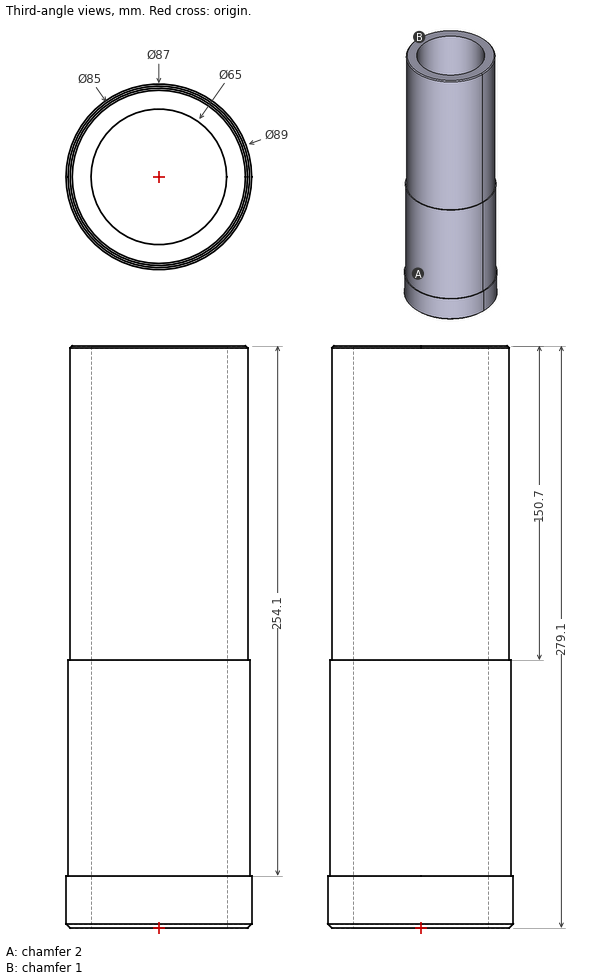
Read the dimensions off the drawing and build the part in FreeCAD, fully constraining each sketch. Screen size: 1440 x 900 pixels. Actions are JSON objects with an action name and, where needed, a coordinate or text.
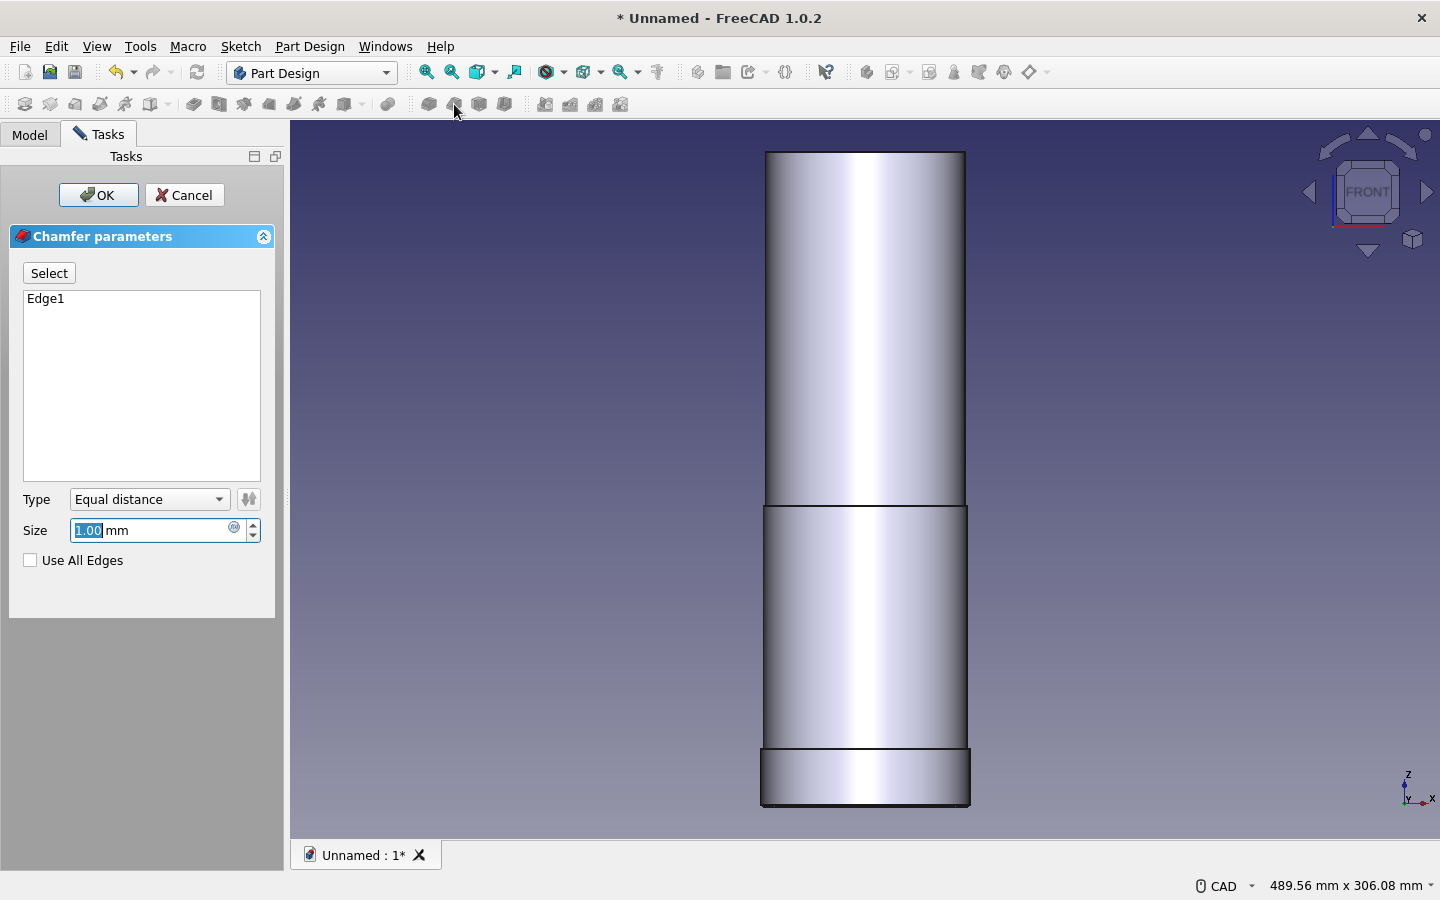
{"action": "type", "text": "2"}
{"action": "key", "text": "Tab"}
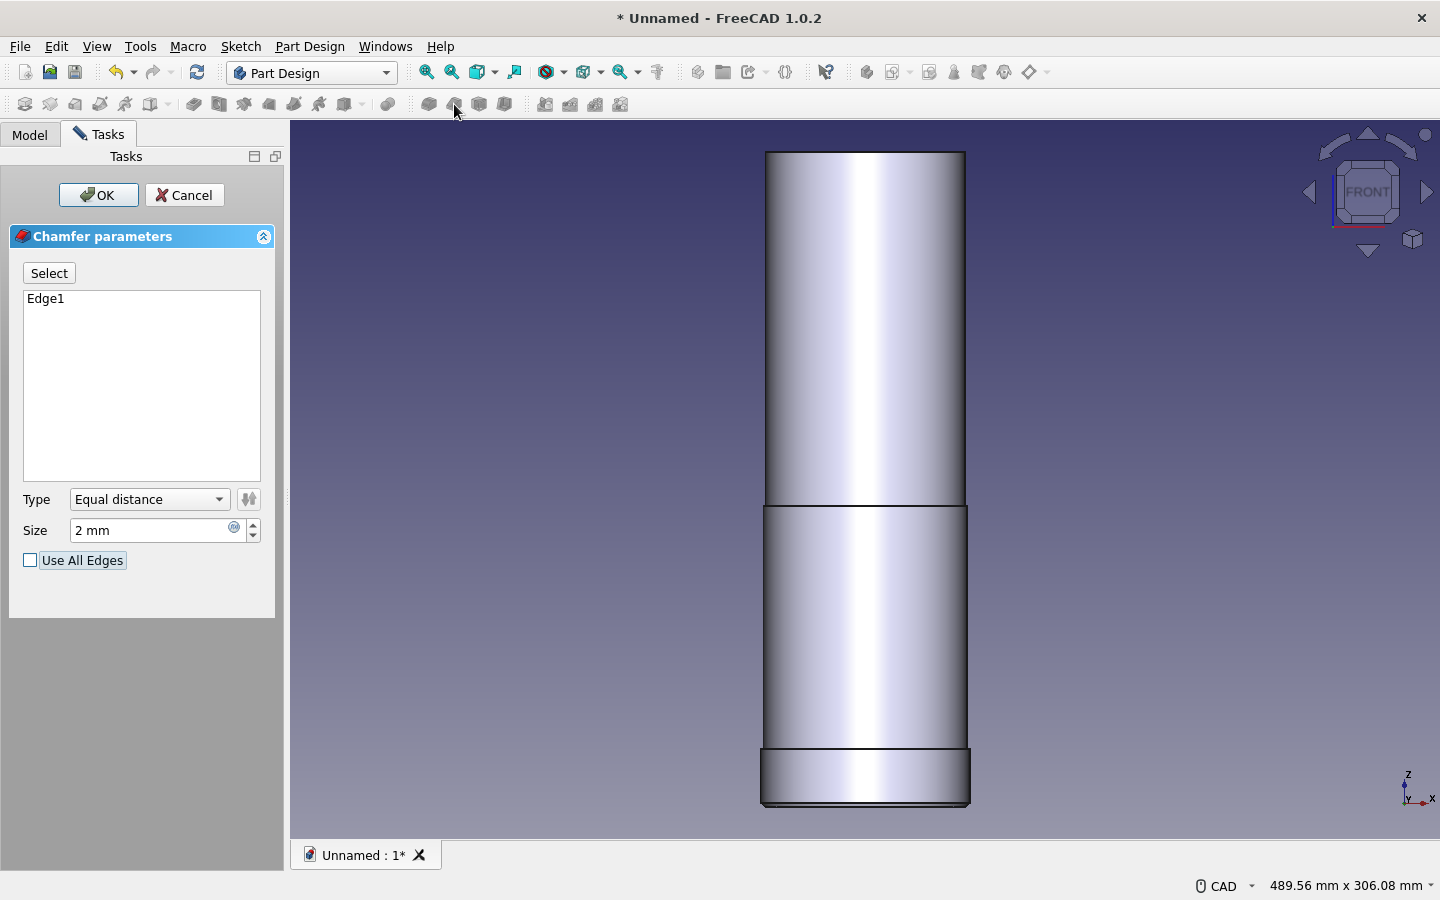
{"action": "left_click", "coordinate": [99, 195]}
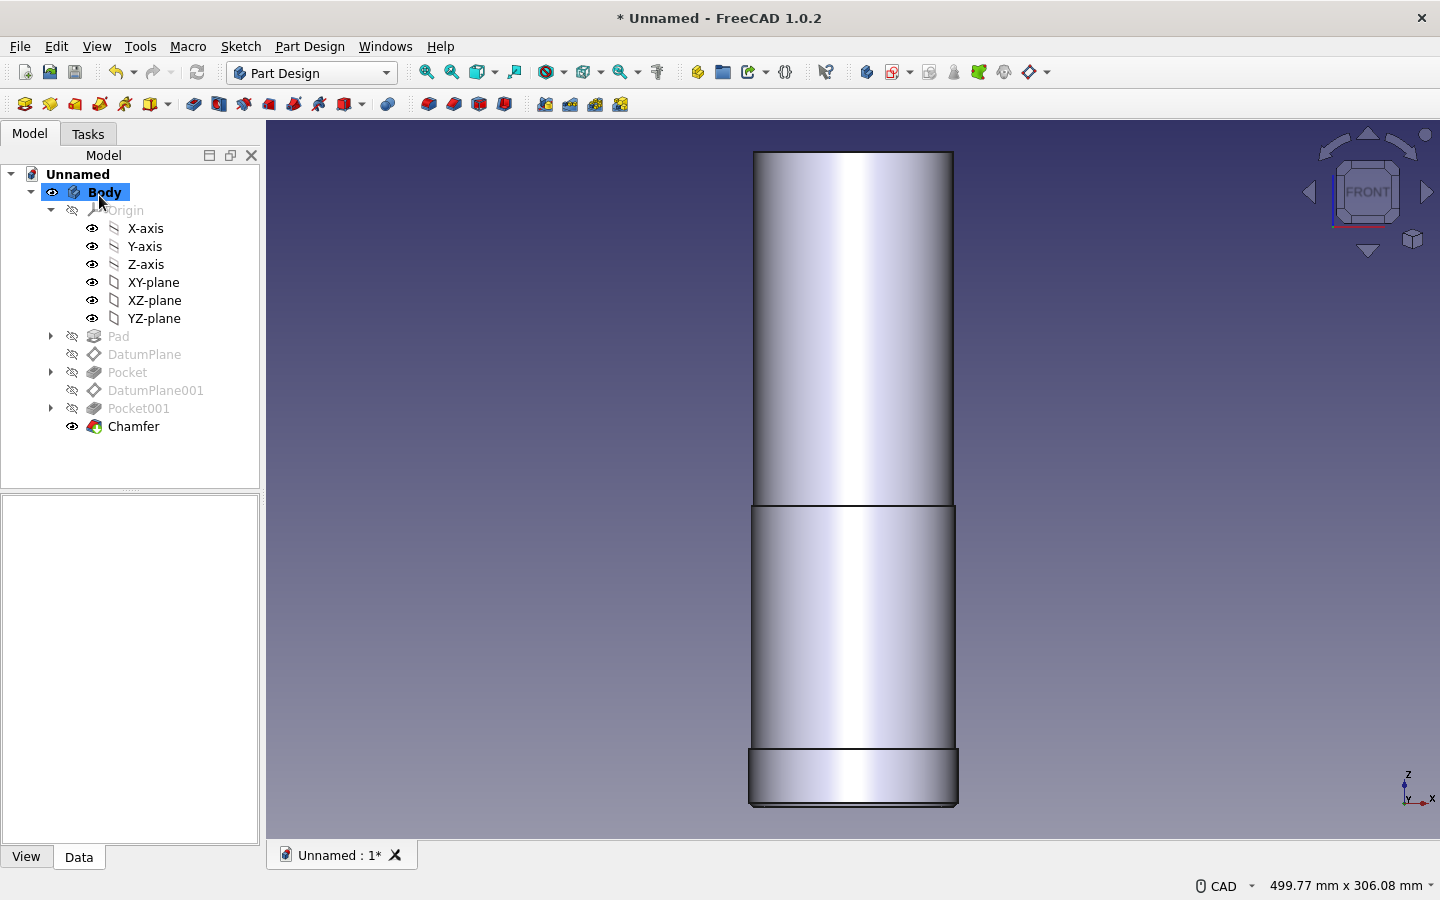
{"action": "left_click", "coordinate": [772, 151]}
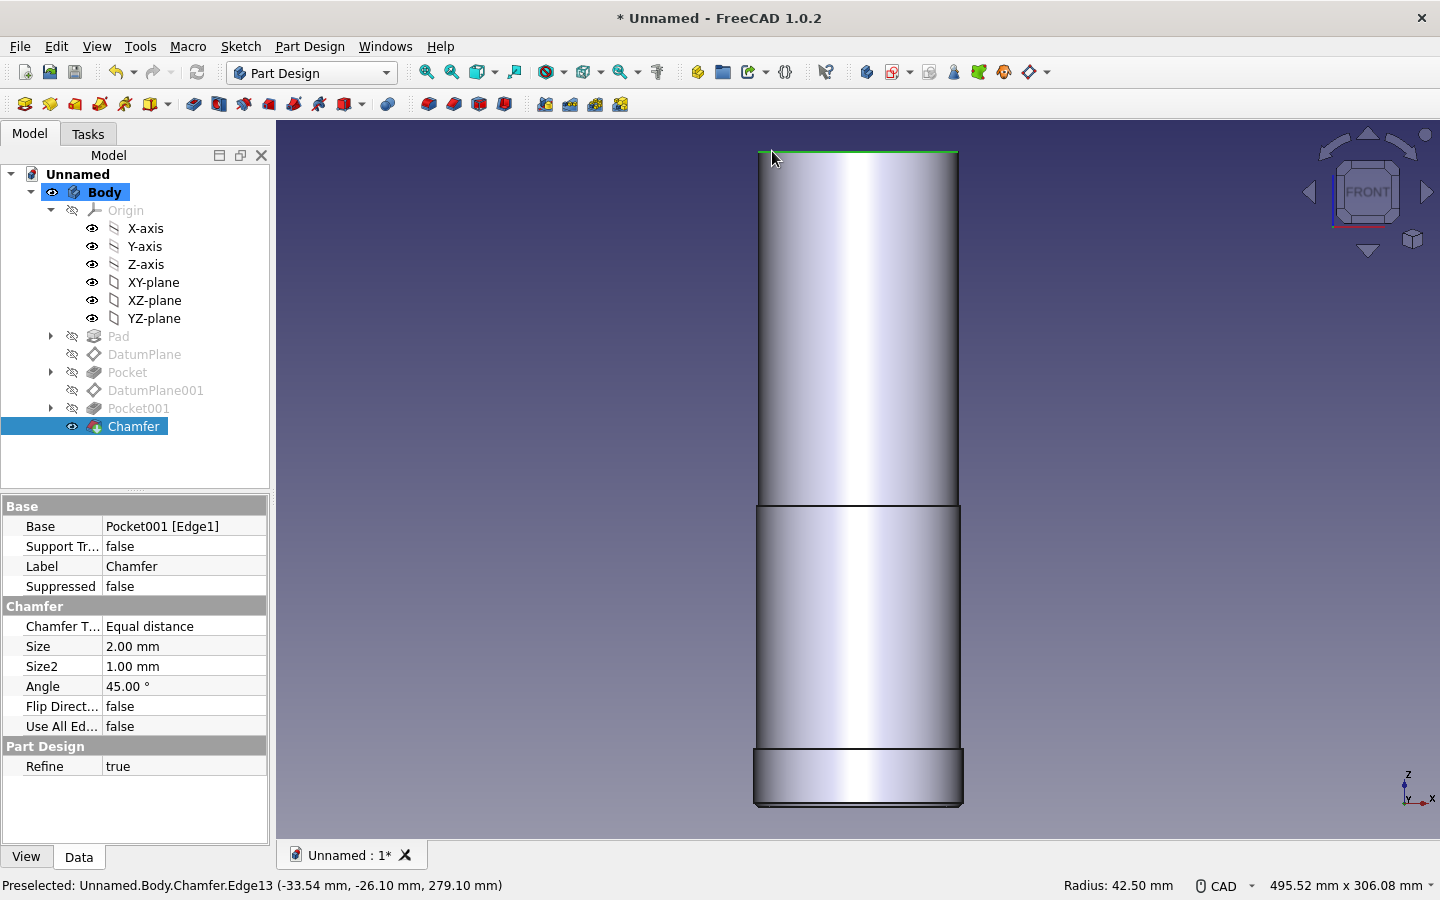
{"action": "left_click", "coordinate": [454, 104]}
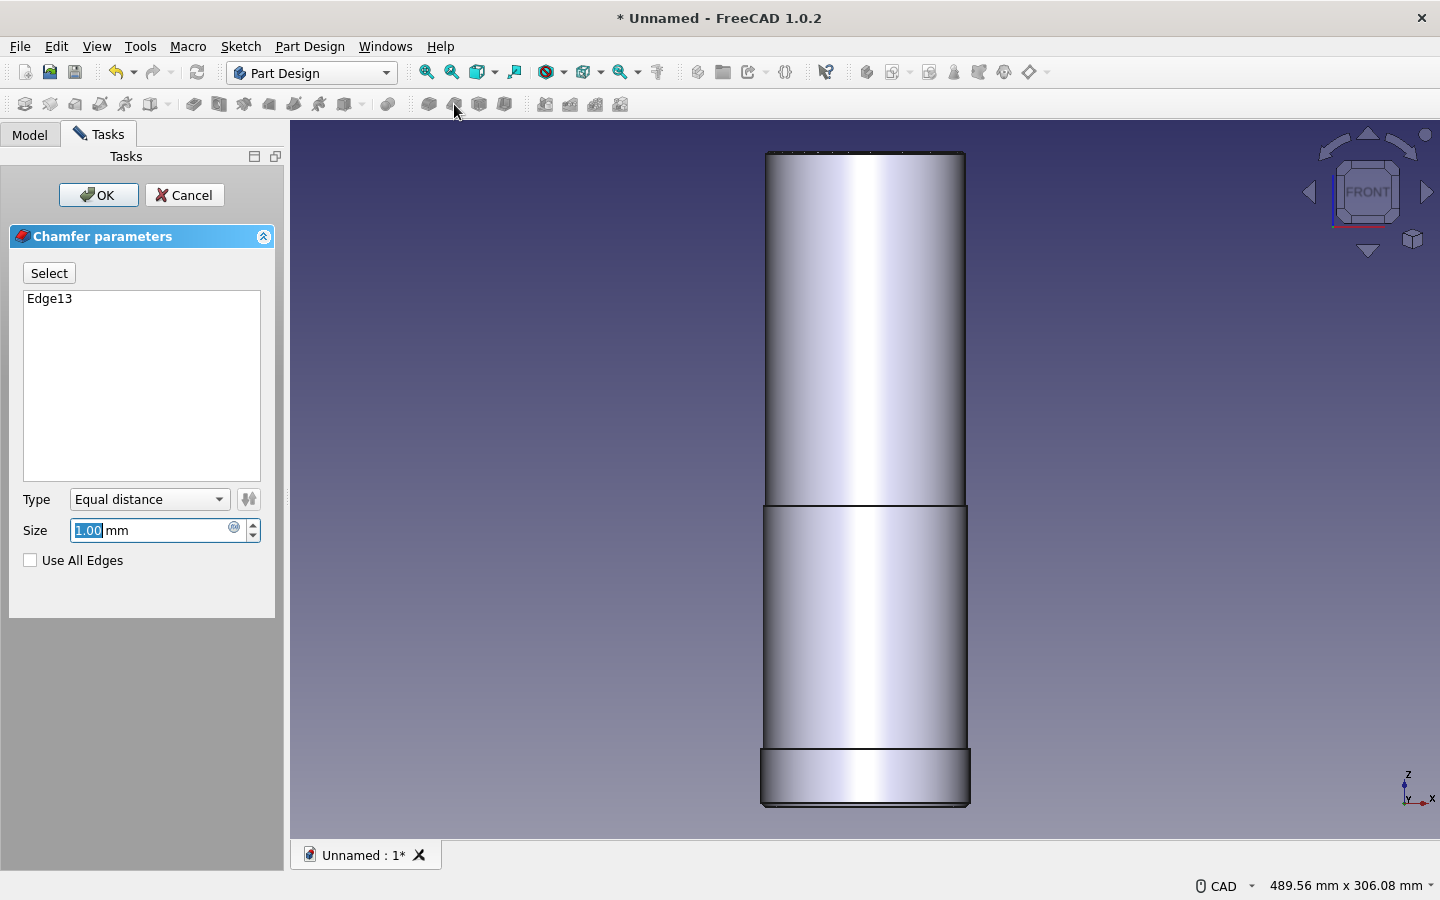
{"action": "type", "text": "1"}
{"action": "key", "text": "Tab"}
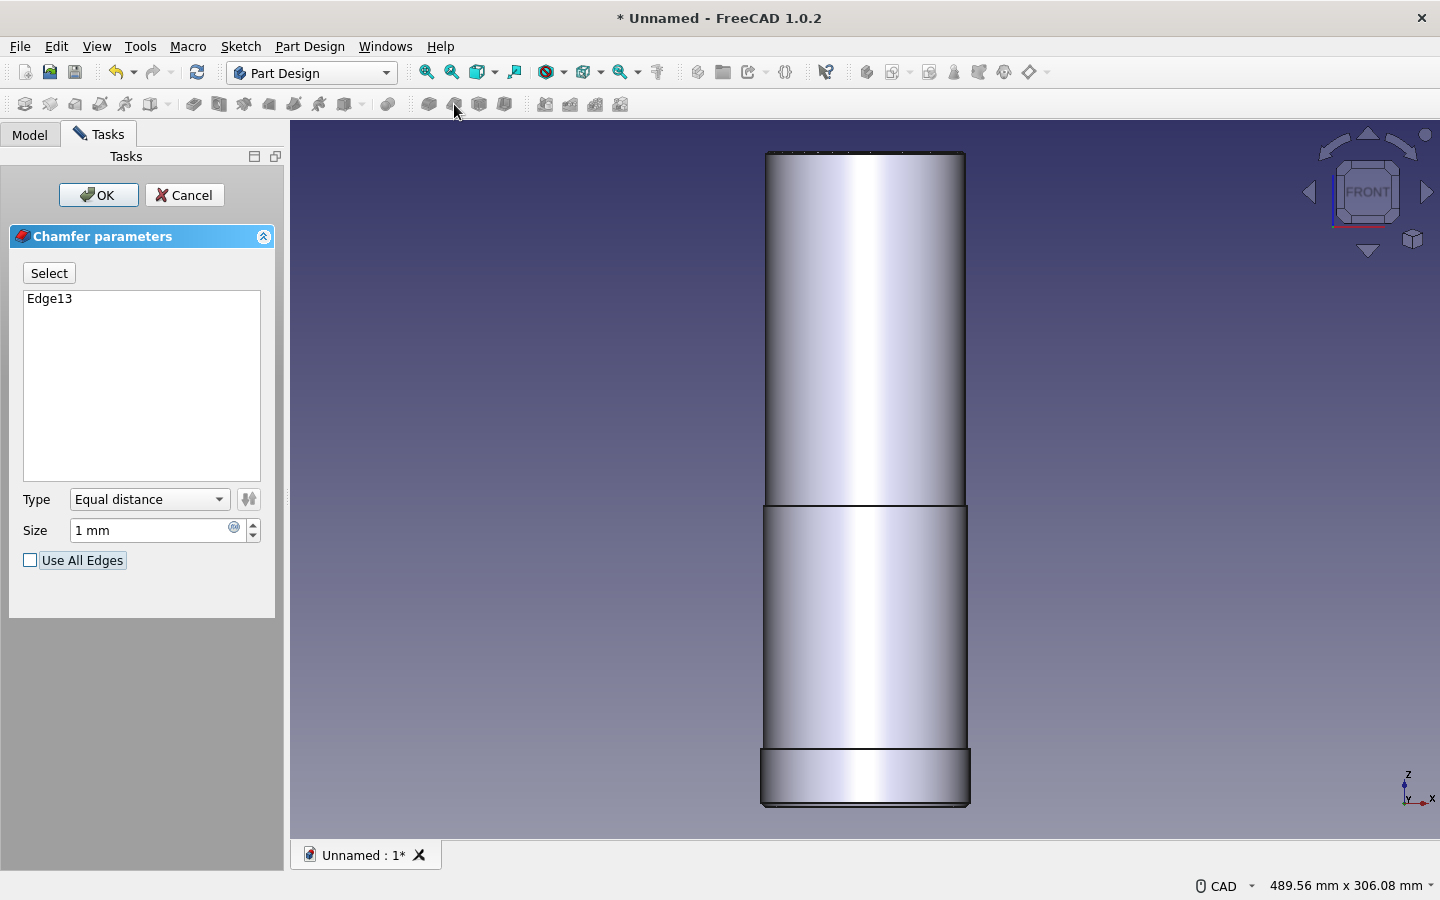
{"action": "left_click", "coordinate": [99, 195]}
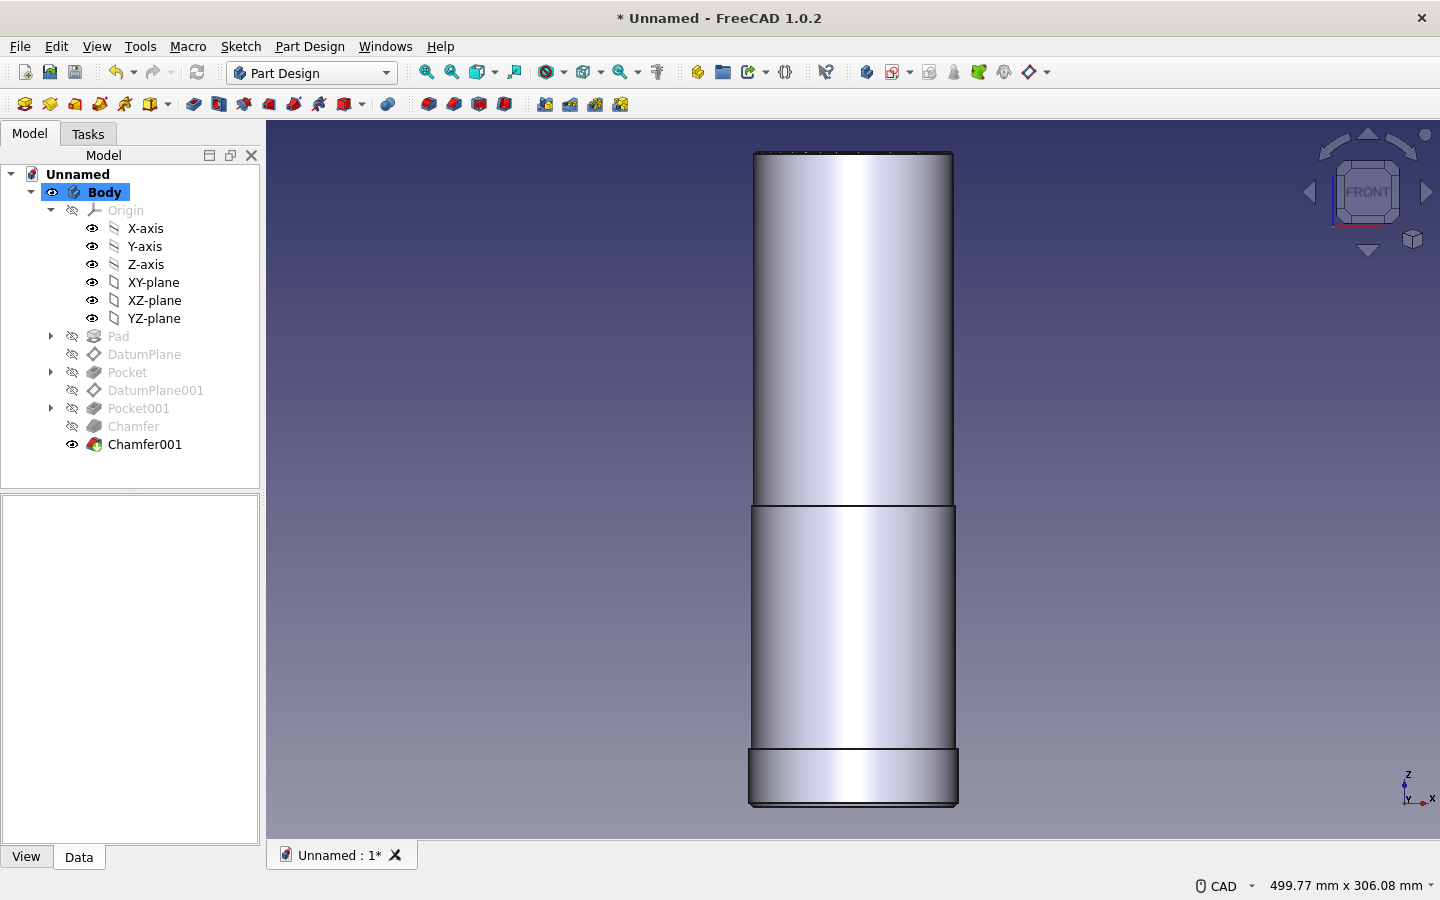
{"action": "key", "text": "0"}